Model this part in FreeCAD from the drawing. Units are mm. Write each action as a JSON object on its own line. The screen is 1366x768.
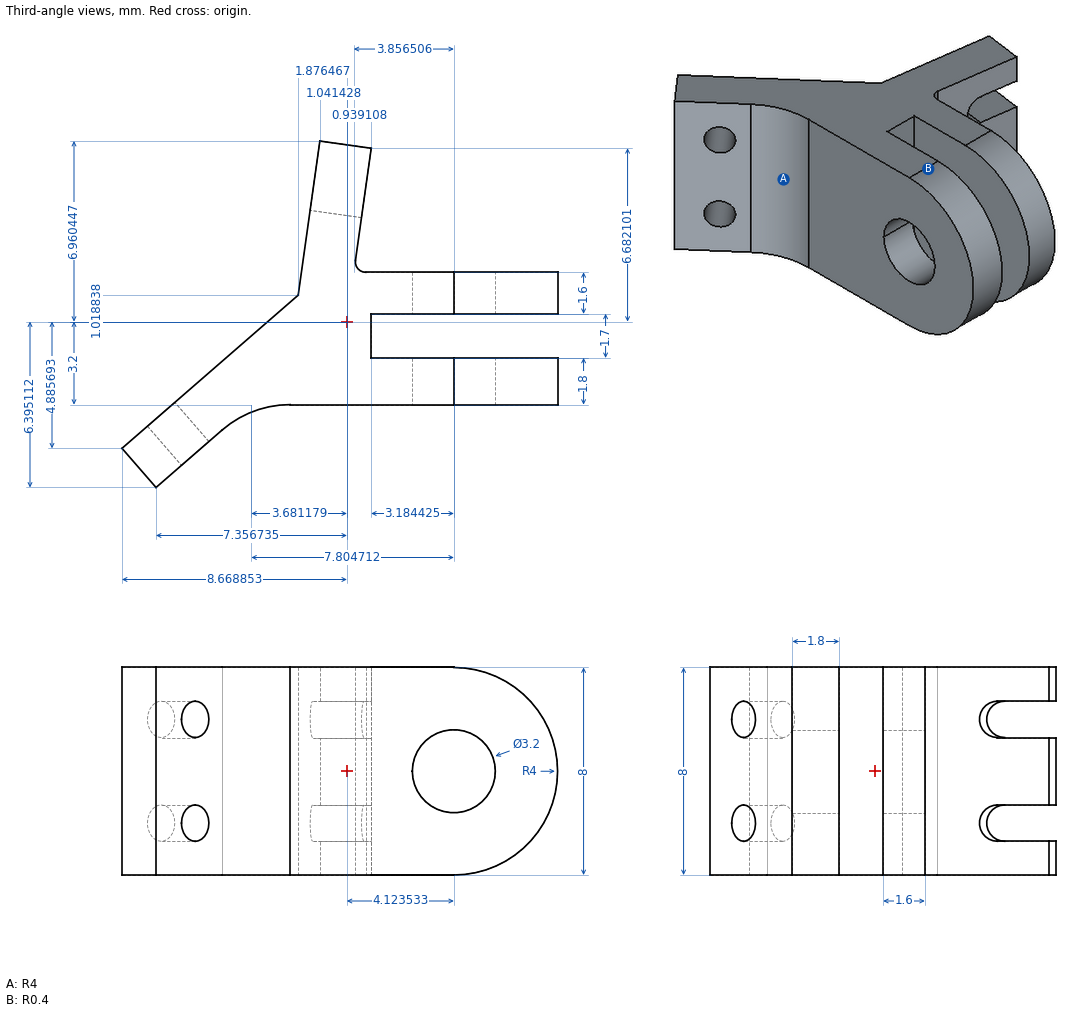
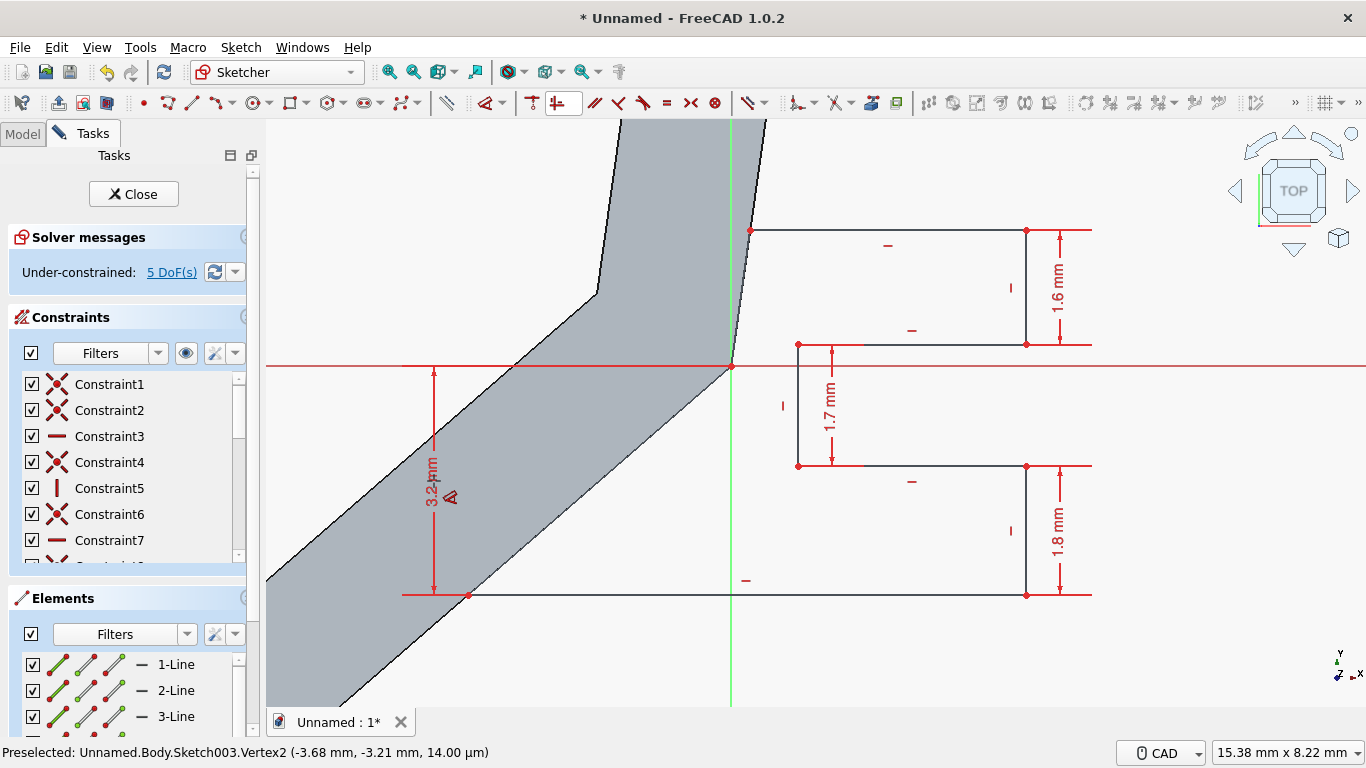
{"action": "left_click", "coordinate": [635, 595]}
{"action": "left_click", "coordinate": [747, 629]}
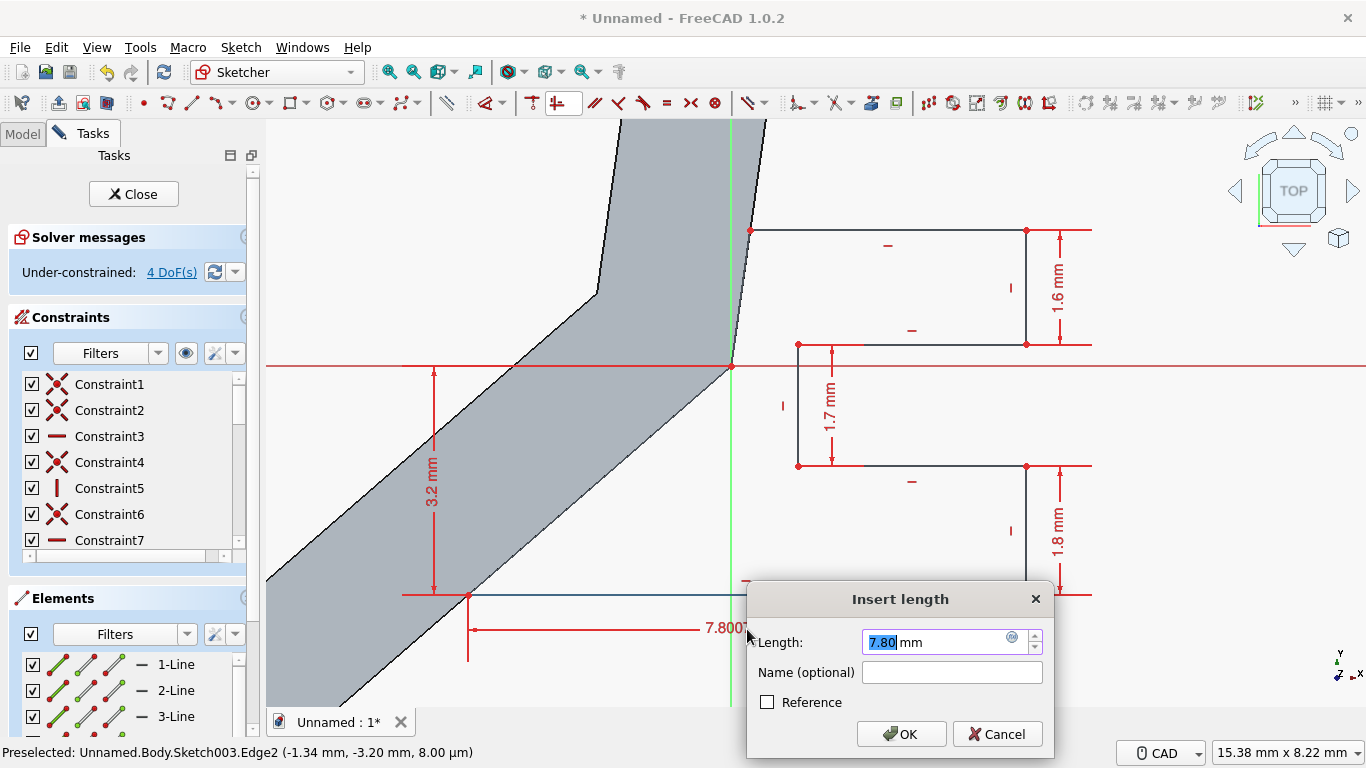
{"action": "type", "text": "7.804712"}
{"action": "key", "text": "Return"}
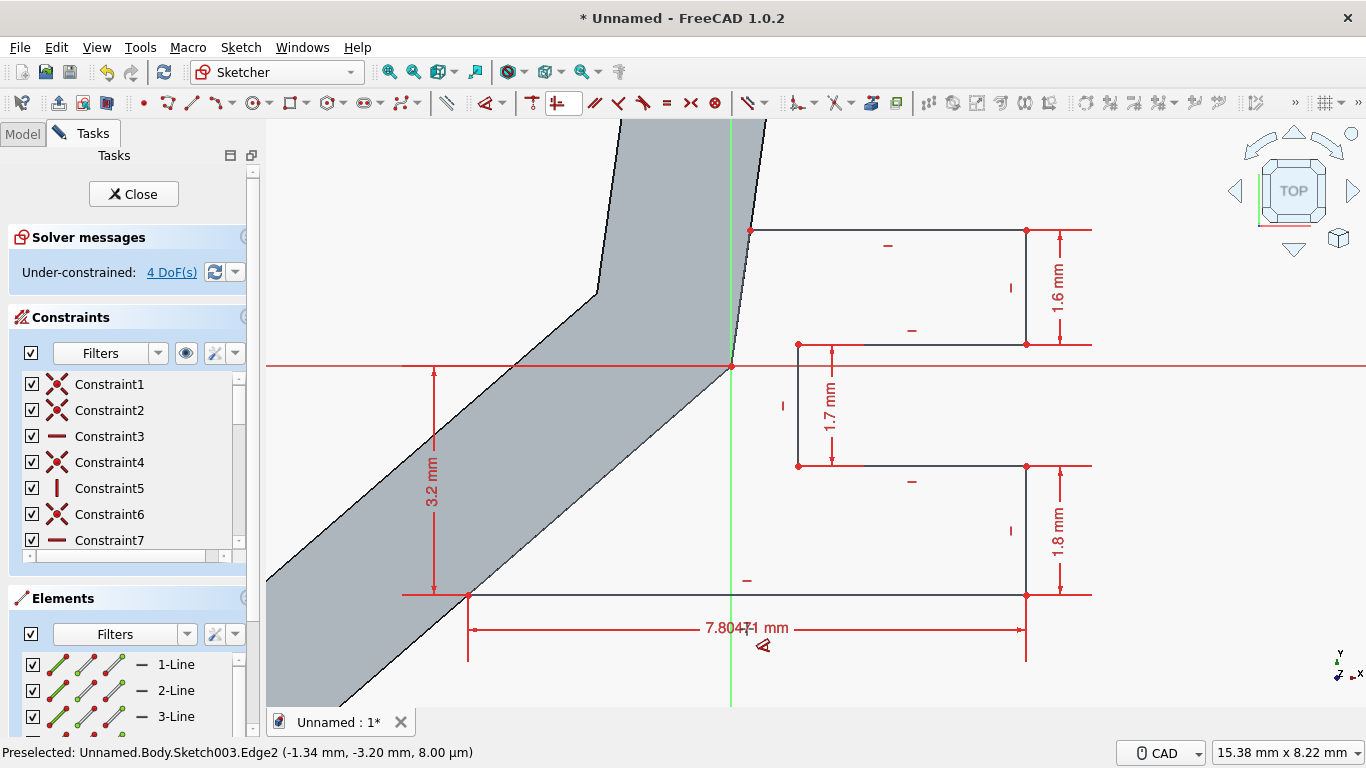
{"action": "left_click", "coordinate": [958, 466]}
{"action": "left_click", "coordinate": [912, 500]}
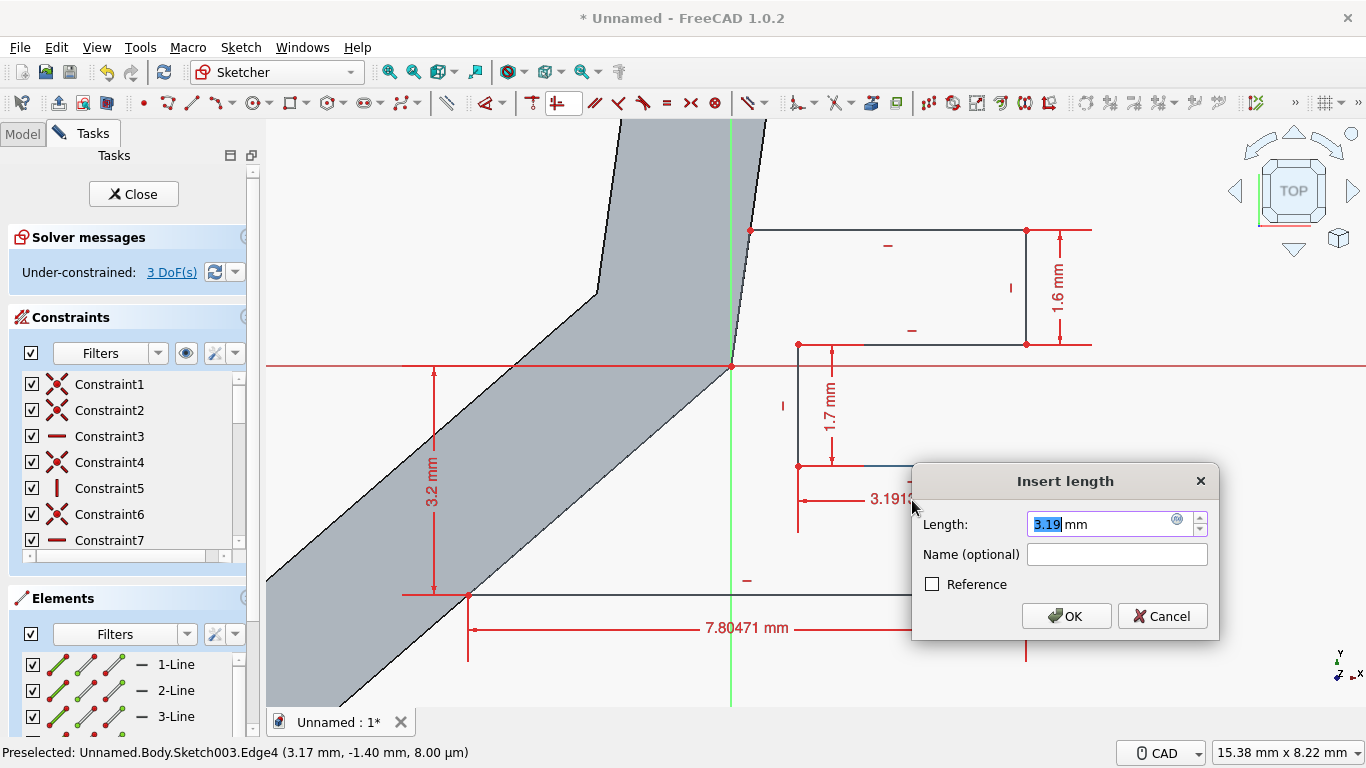
{"action": "type", "text": "3.184425"}
{"action": "key", "text": "Return"}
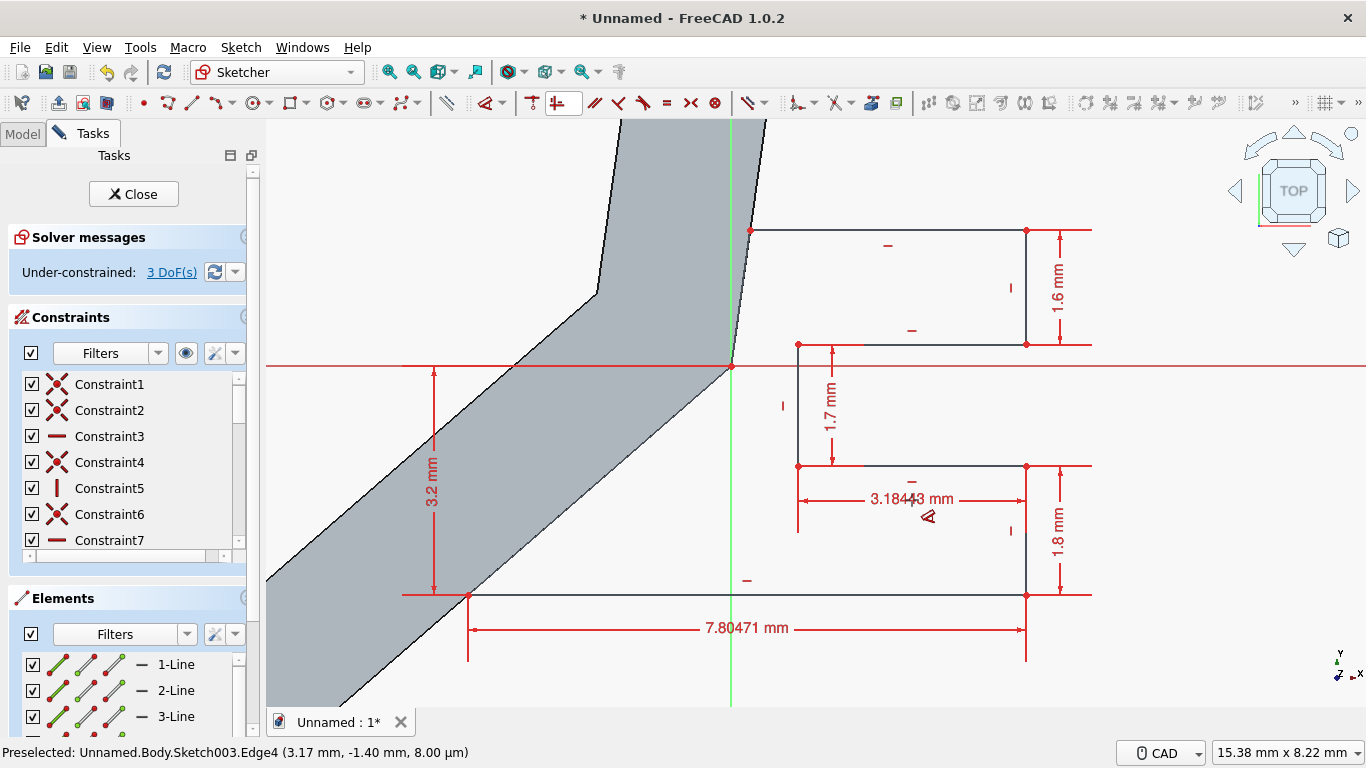
{"action": "left_click", "coordinate": [867, 345]}
{"action": "left_click", "coordinate": [912, 311]}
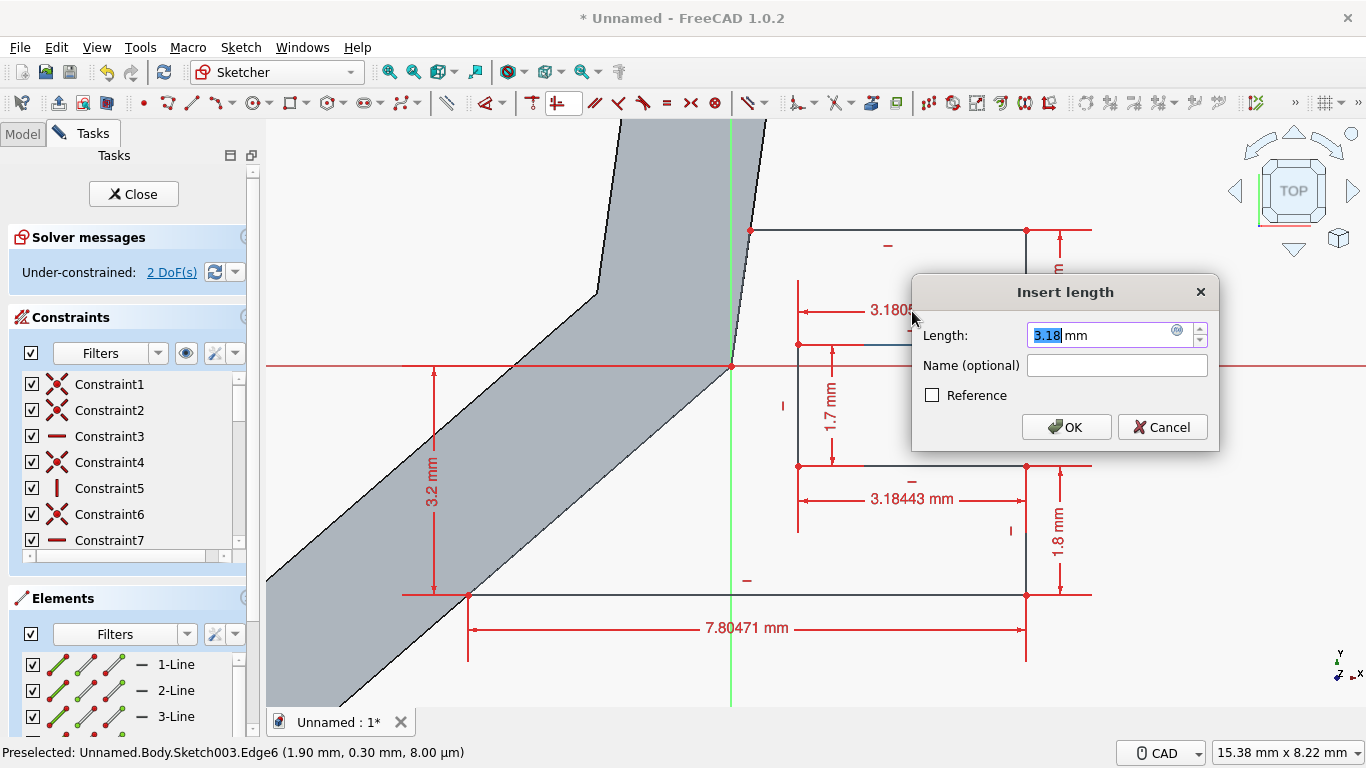
{"action": "type", "text": "3.184425"}
{"action": "key", "text": "Return"}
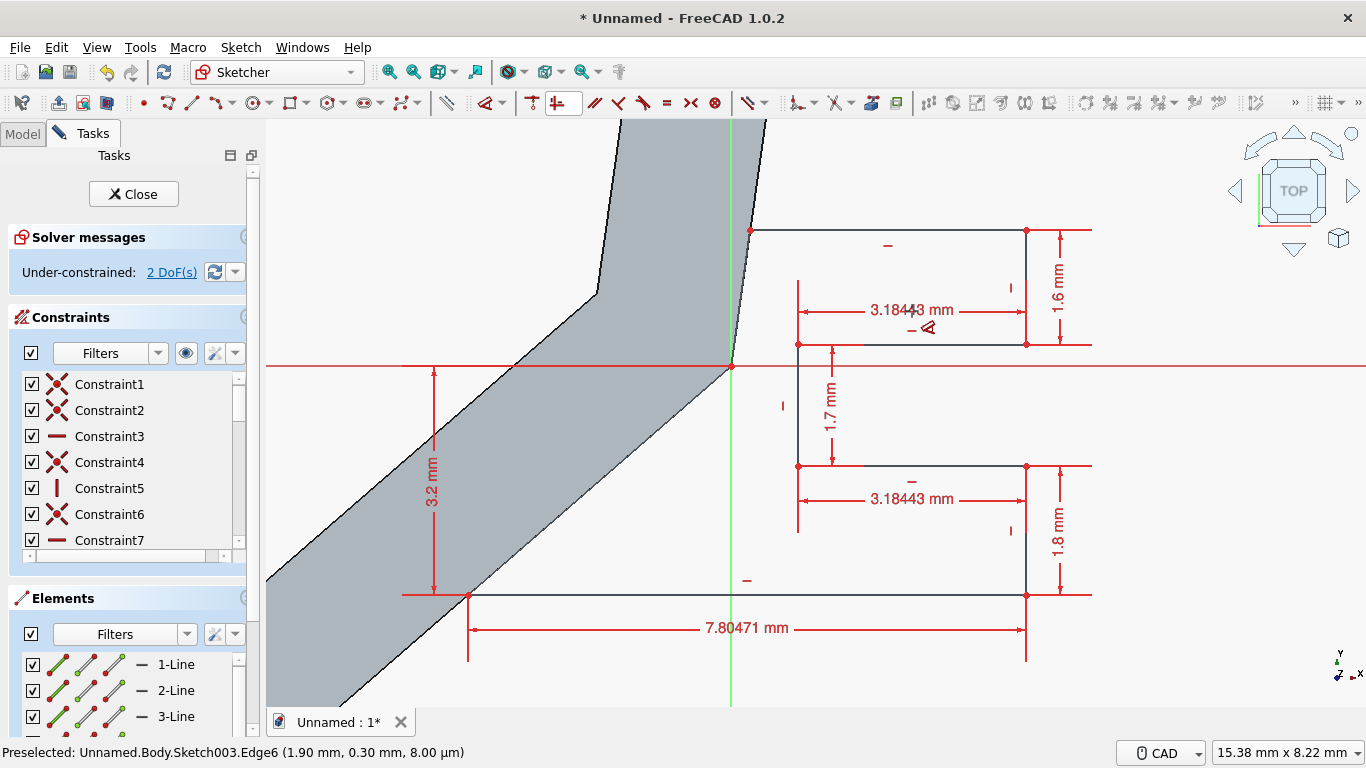
{"action": "left_click", "coordinate": [943, 230]}
{"action": "left_click", "coordinate": [888, 196]}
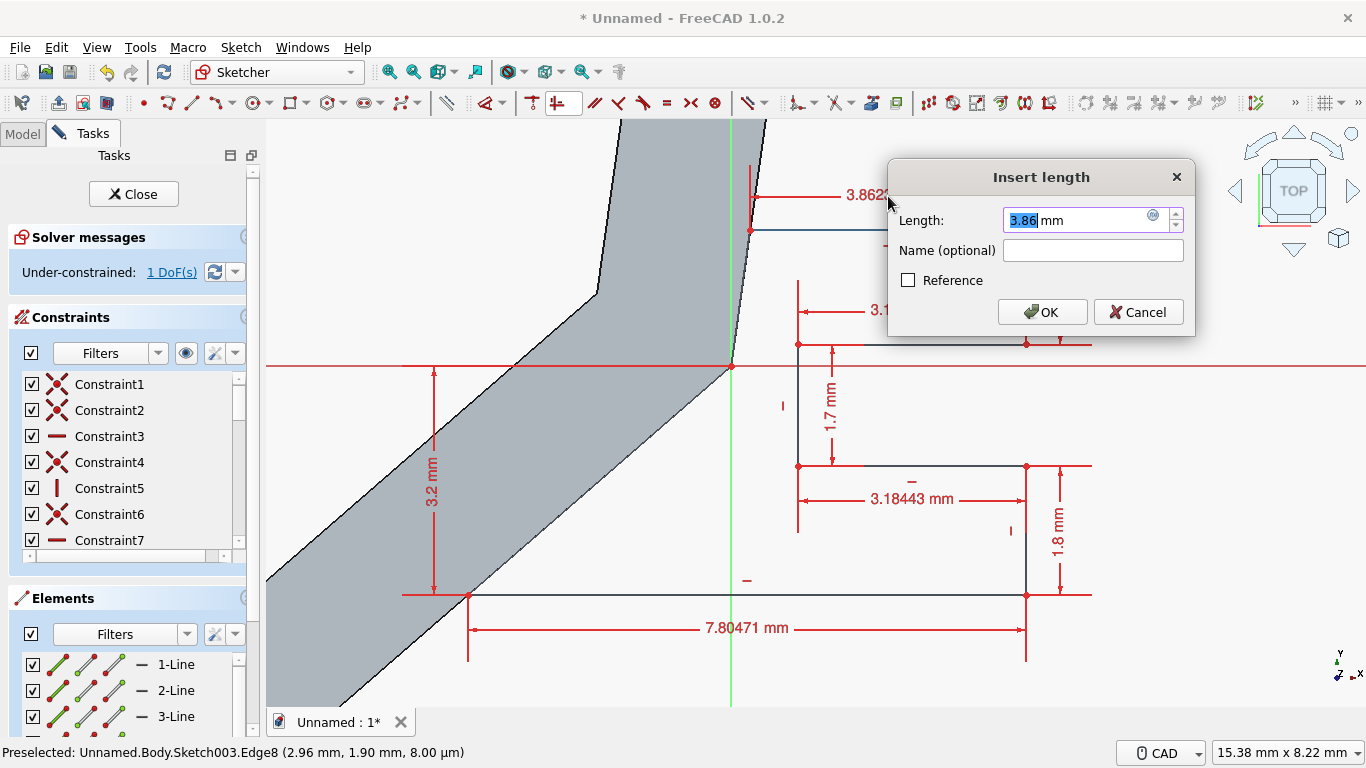
{"action": "type", "text": "3.856506"}
{"action": "key", "text": "Return"}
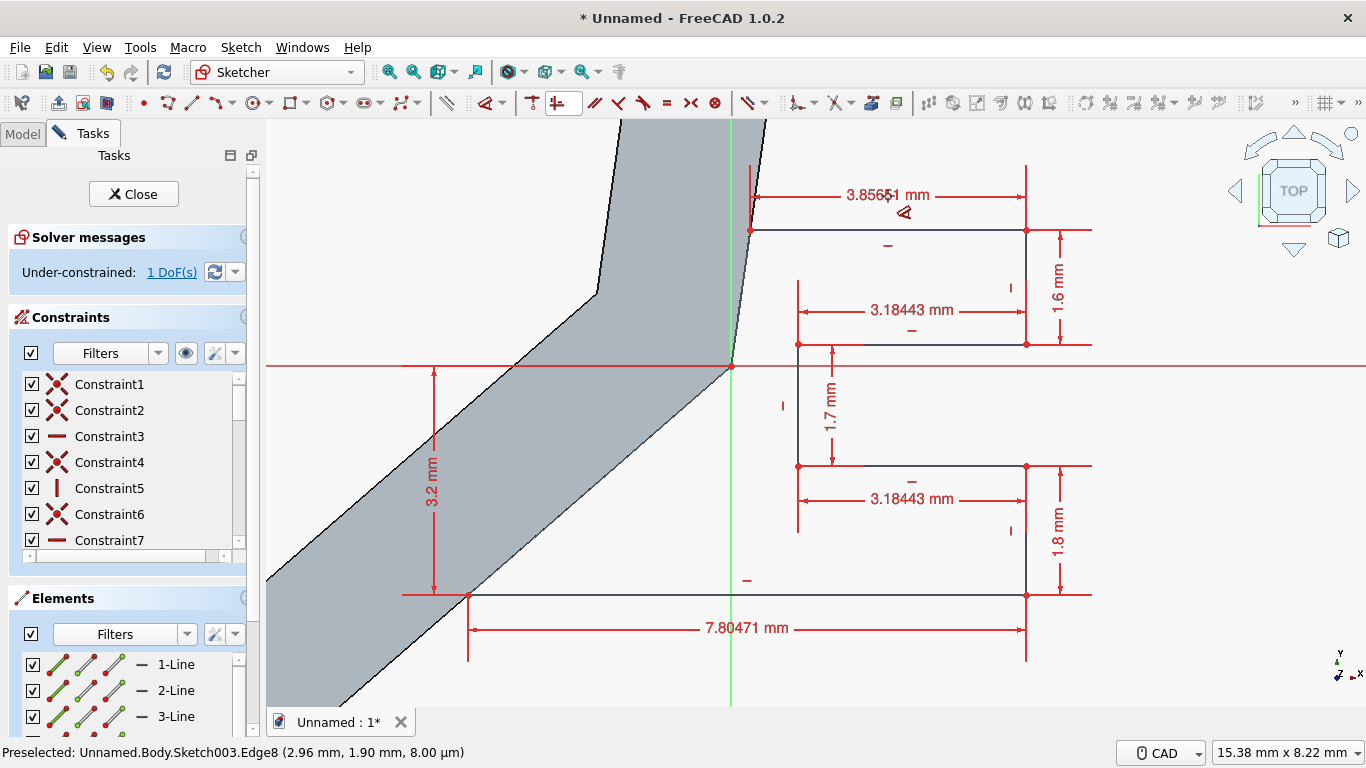
{"action": "left_click", "coordinate": [468, 595]}
{"action": "left_click", "coordinate": [600, 629]}